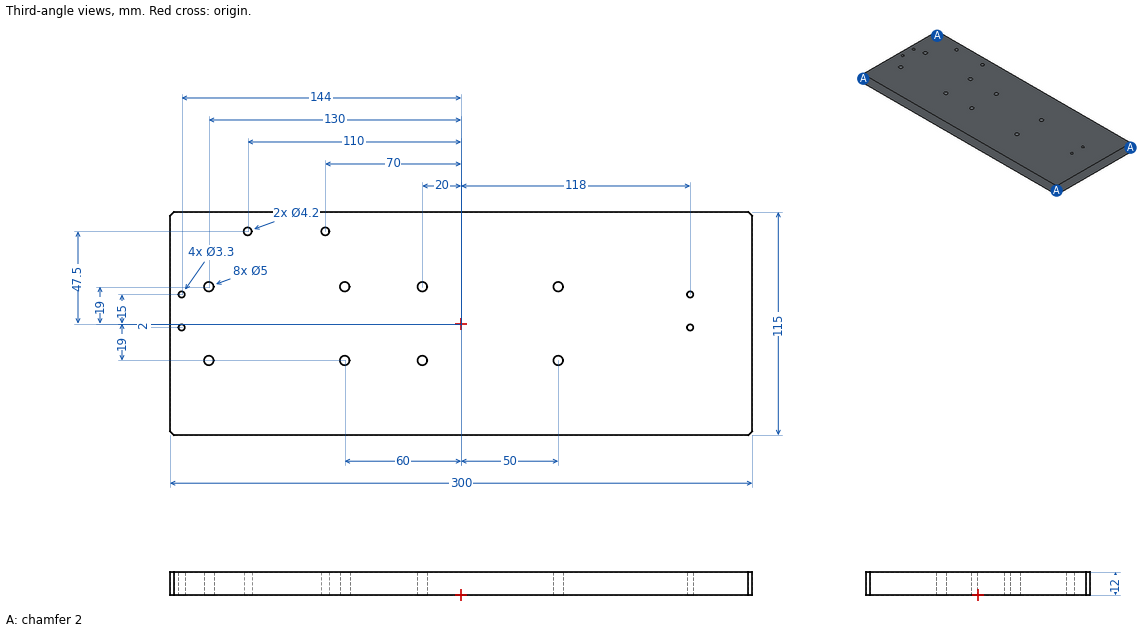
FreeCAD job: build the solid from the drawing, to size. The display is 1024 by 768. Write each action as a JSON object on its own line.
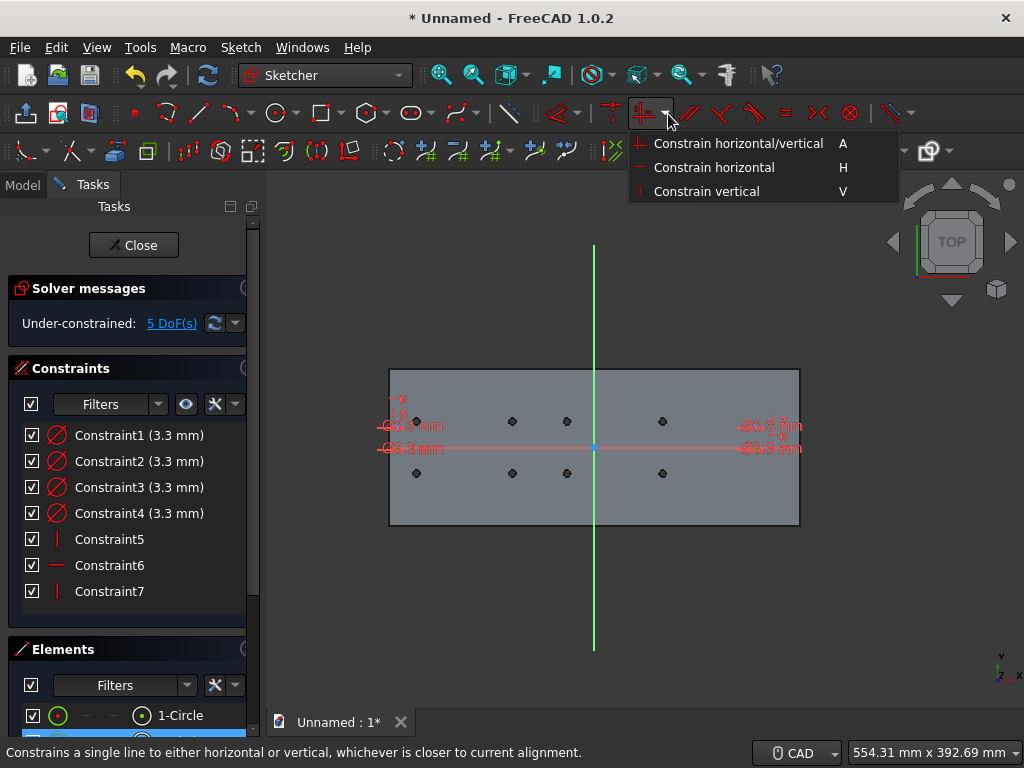
{"action": "left_click", "coordinate": [764, 167]}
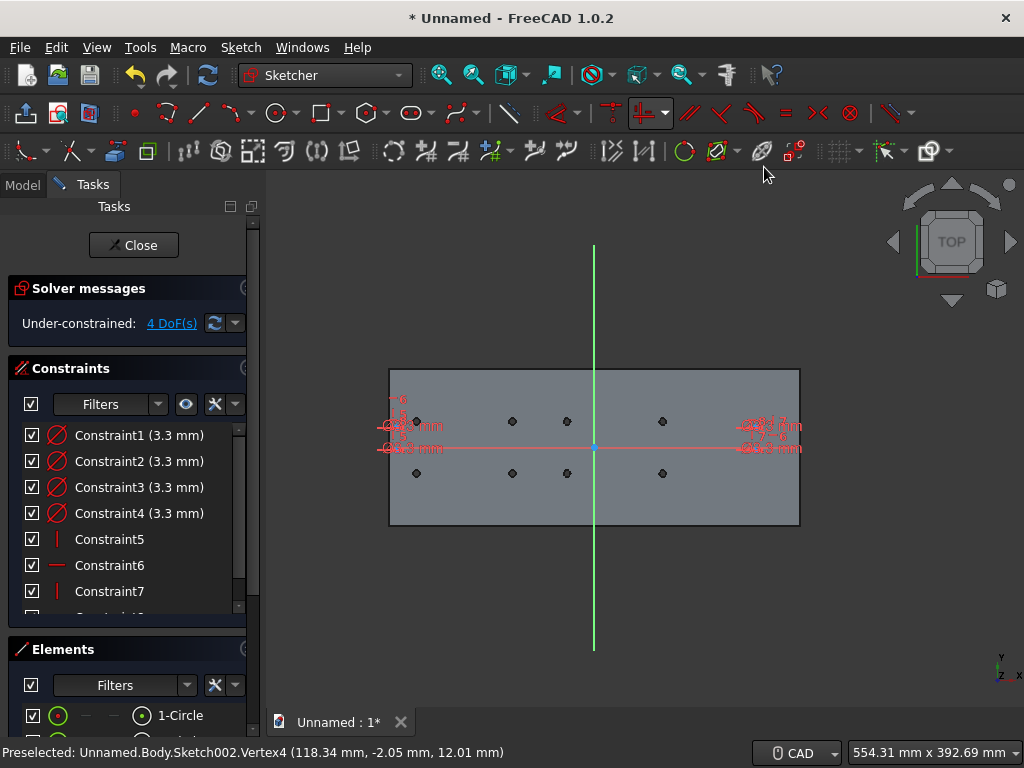
{"action": "left_click", "coordinate": [556, 114]}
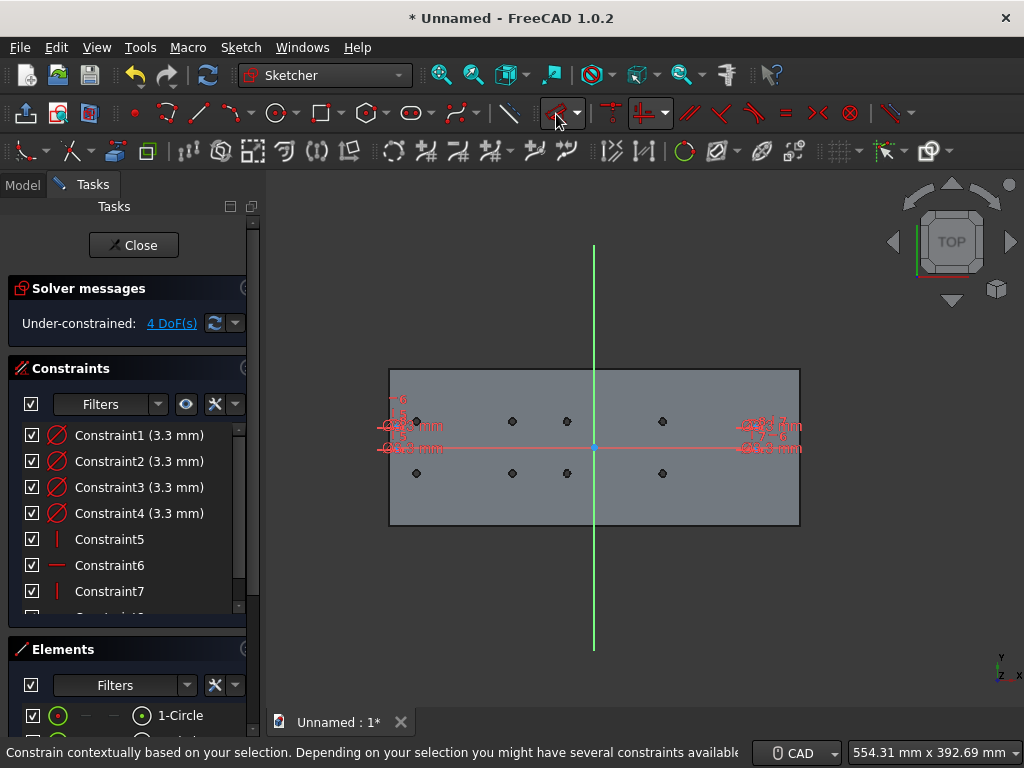
{"action": "scroll", "coordinate": [397, 450], "scroll_direction": "up", "scroll_amount": 14}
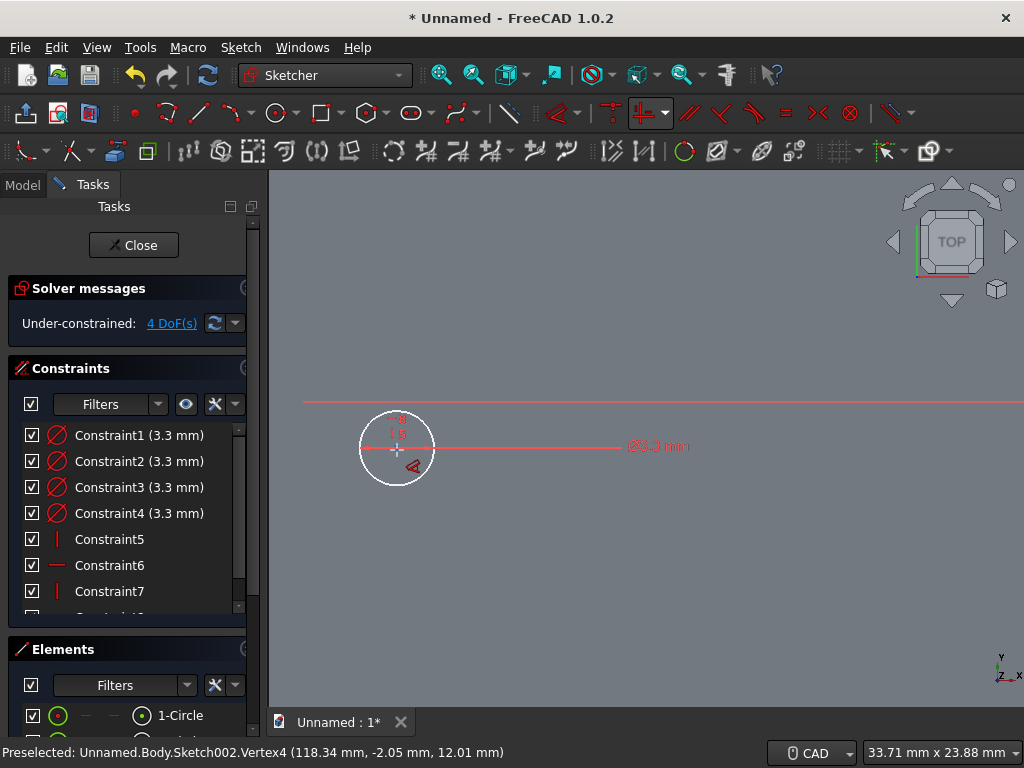
{"action": "left_click", "coordinate": [397, 448]}
{"action": "left_click", "coordinate": [339, 425]}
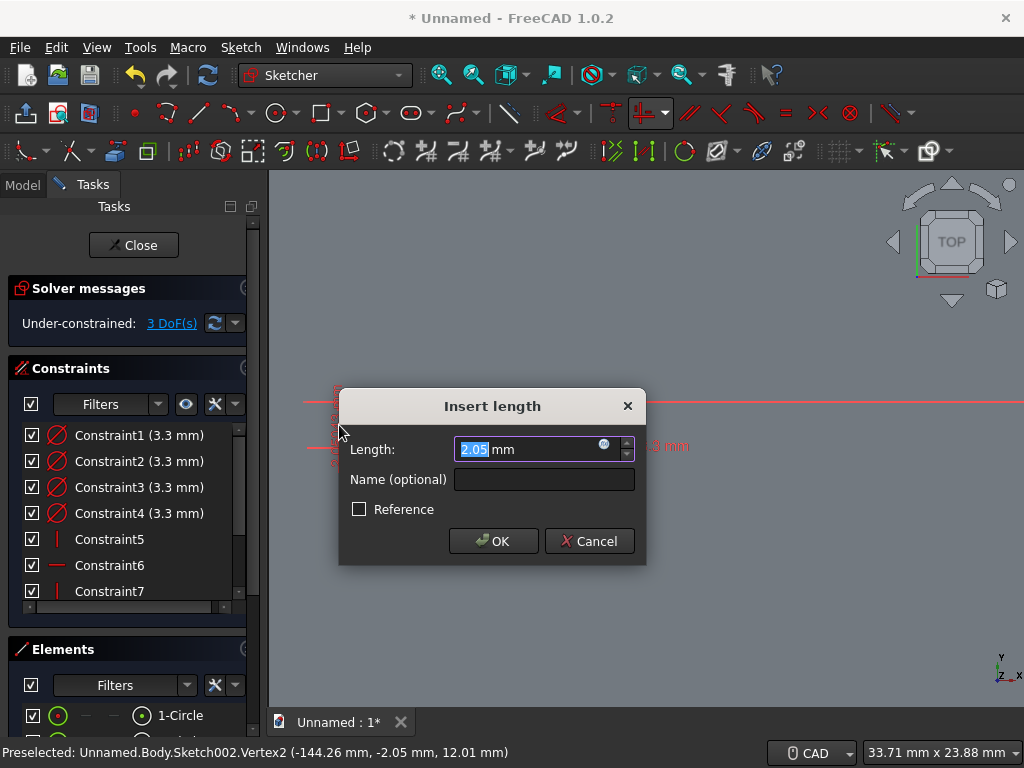
{"action": "type", "text": "2"}
{"action": "key", "text": "Return"}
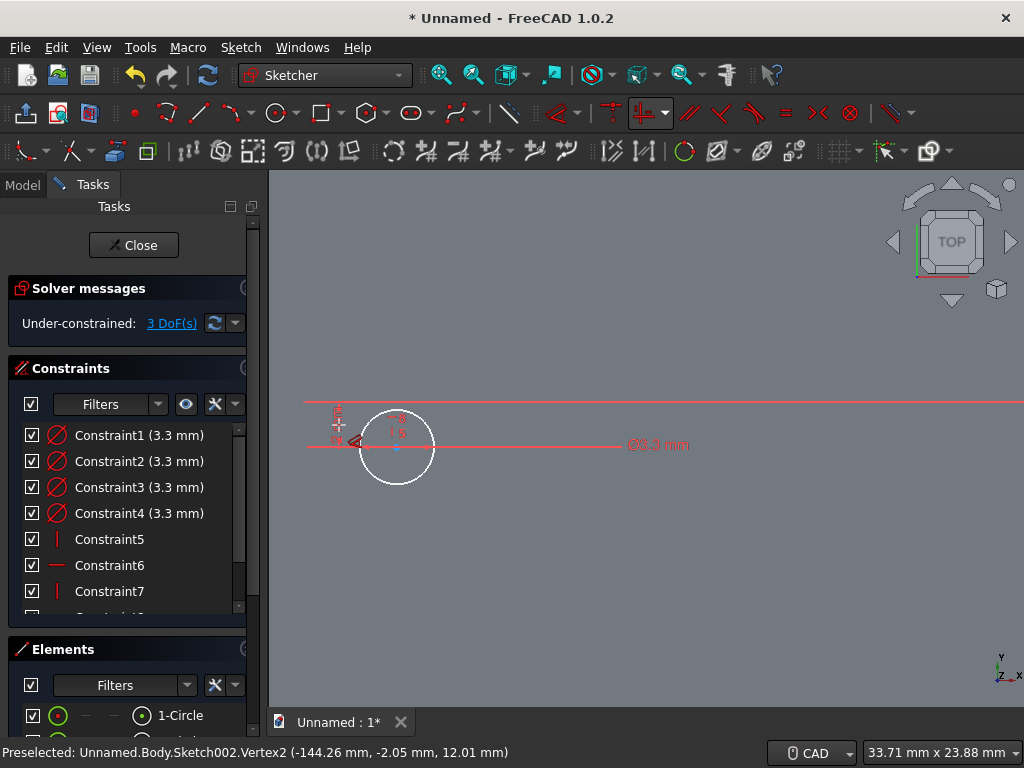
{"action": "scroll", "coordinate": [397, 450], "scroll_direction": "down", "scroll_amount": 14}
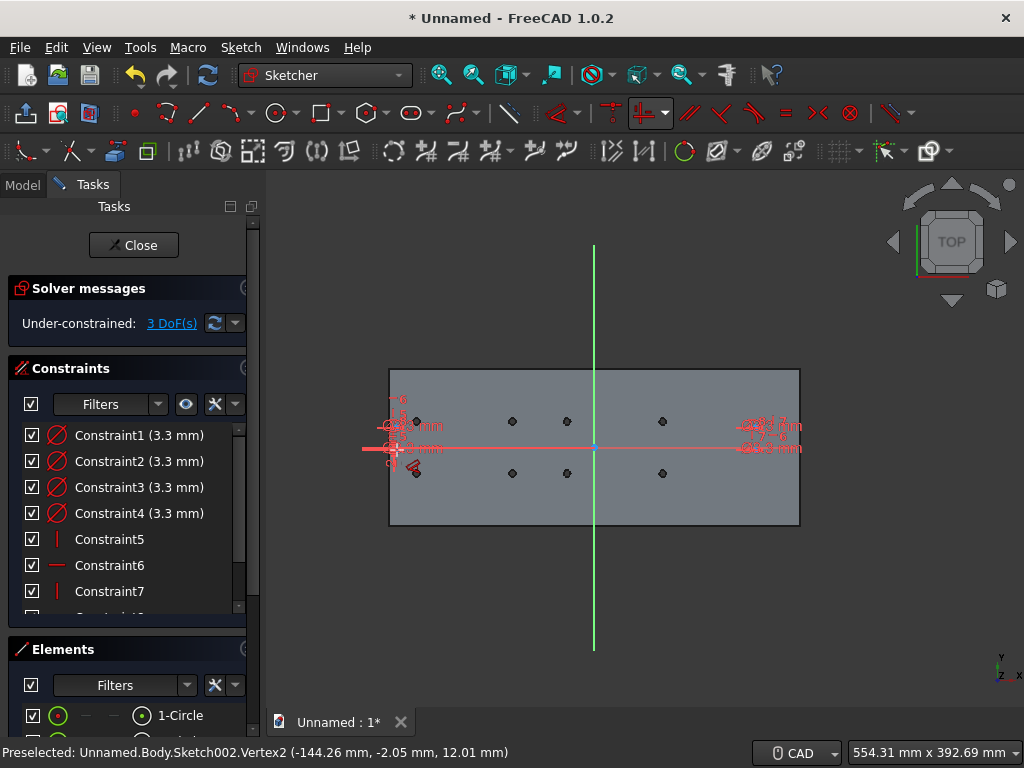
{"action": "scroll", "coordinate": [397, 428], "scroll_direction": "up", "scroll_amount": 4}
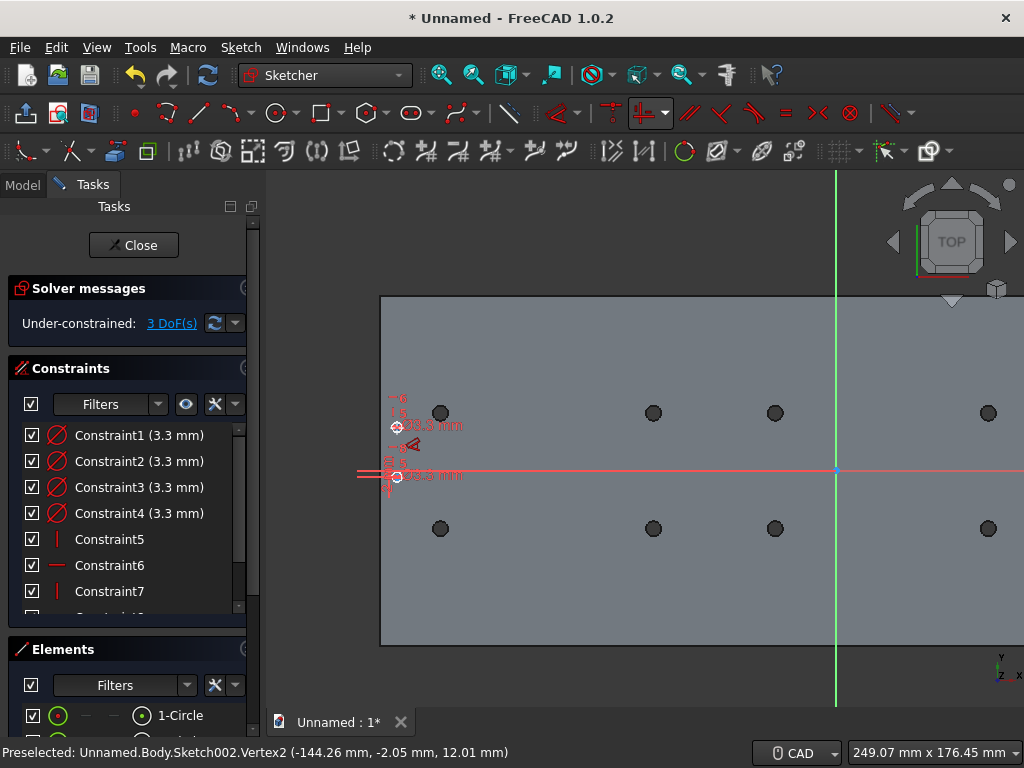
{"action": "left_click", "coordinate": [397, 427]}
{"action": "left_click", "coordinate": [363, 449]}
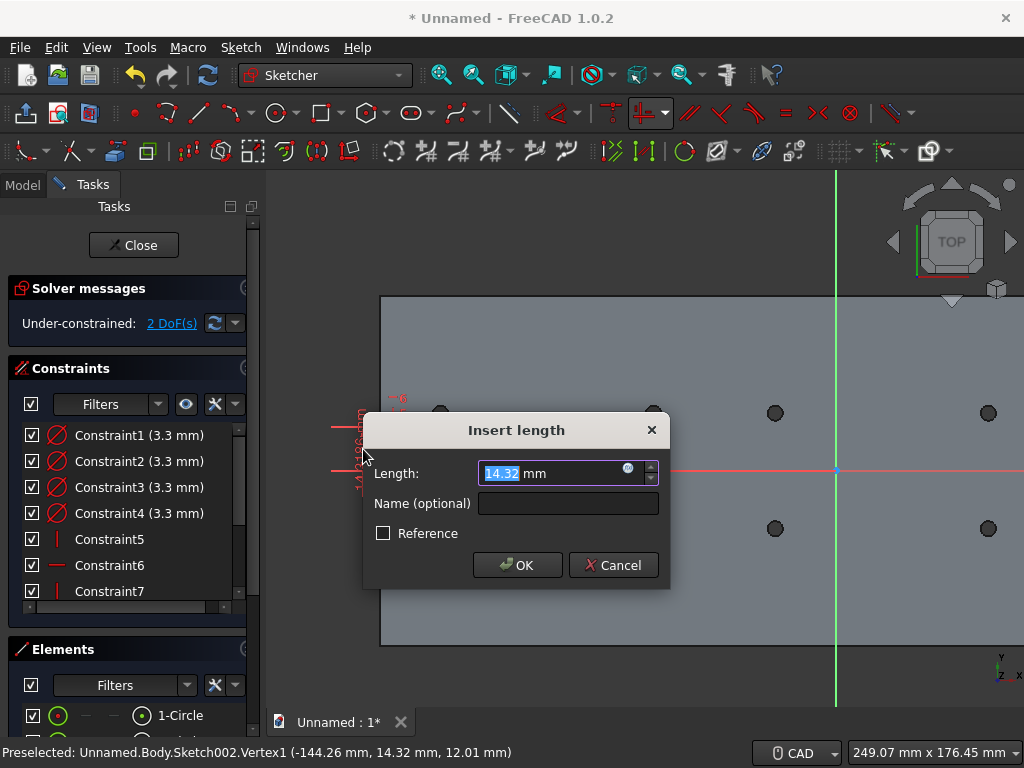
{"action": "type", "text": "15"}
{"action": "key", "text": "Return"}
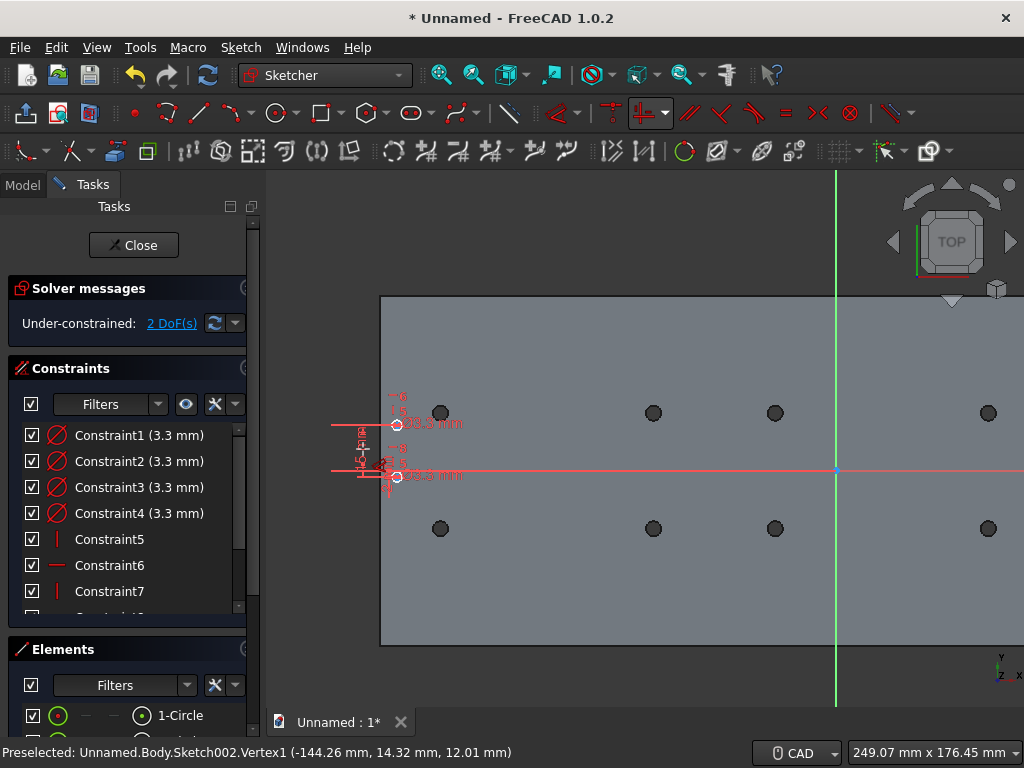
{"action": "left_click", "coordinate": [397, 425]}
{"action": "left_click", "coordinate": [617, 391]}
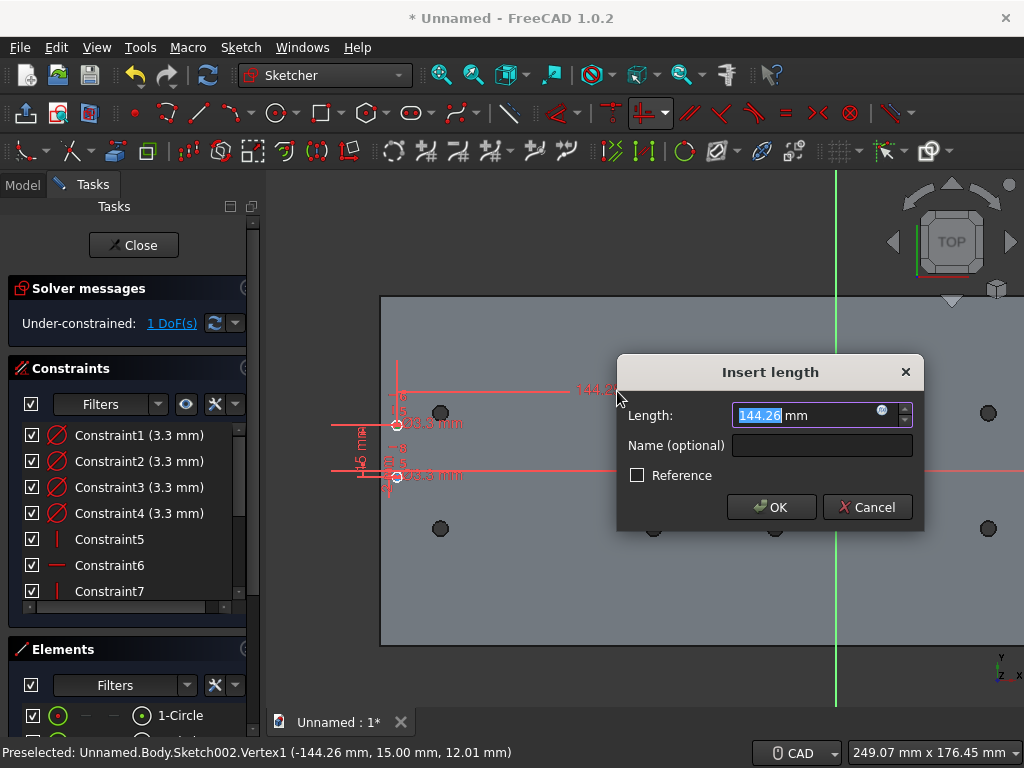
{"action": "type", "text": "144"}
{"action": "key", "text": "Return"}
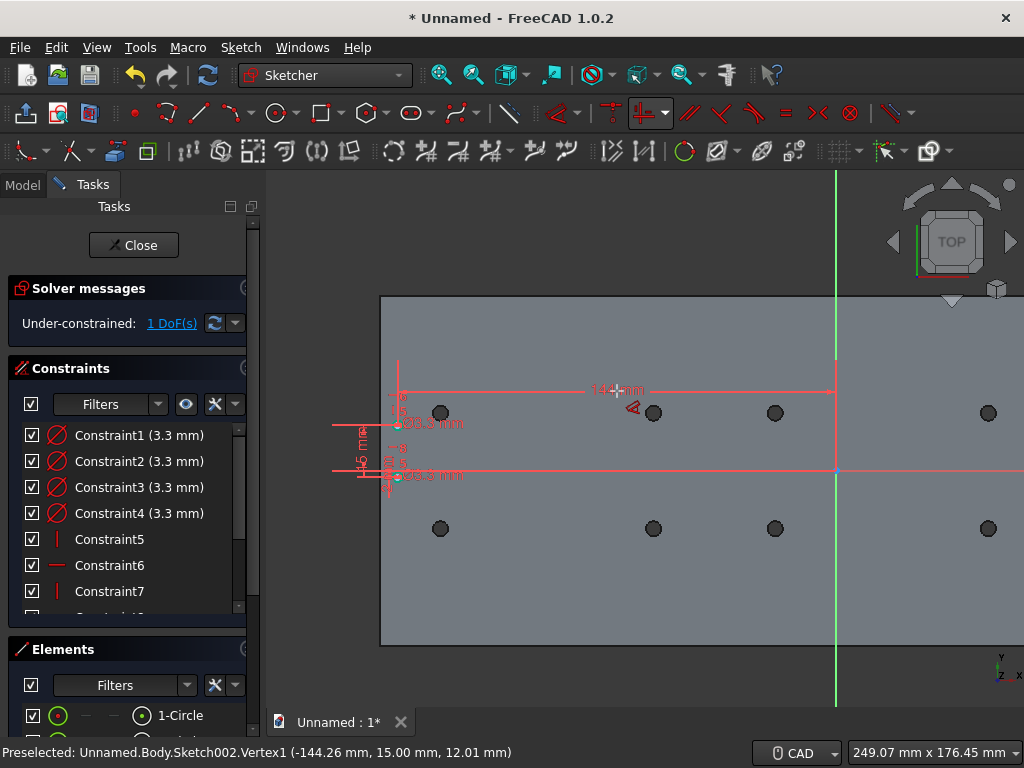
{"action": "scroll", "coordinate": [397, 428], "scroll_direction": "down", "scroll_amount": 4}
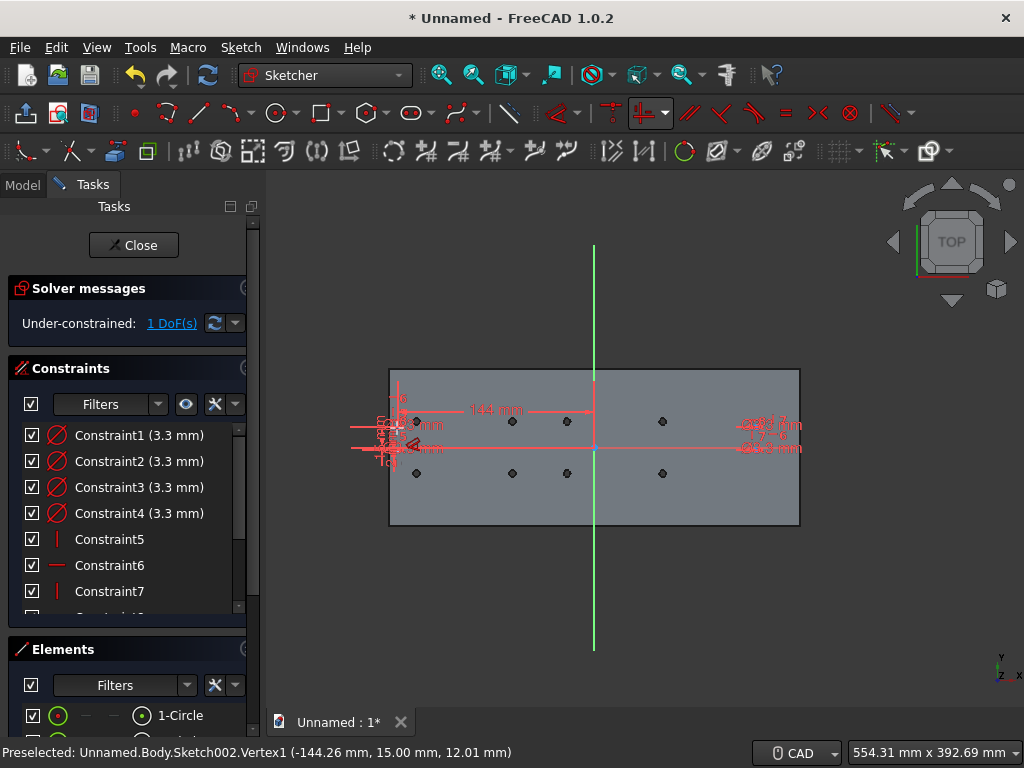
{"action": "left_click", "coordinate": [756, 427]}
{"action": "left_click", "coordinate": [675, 393]}